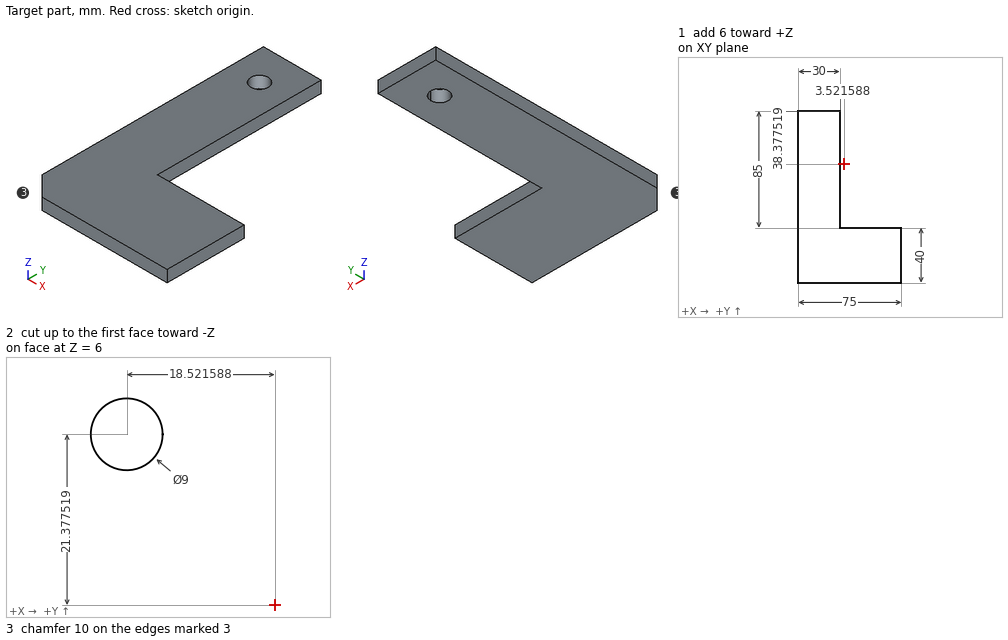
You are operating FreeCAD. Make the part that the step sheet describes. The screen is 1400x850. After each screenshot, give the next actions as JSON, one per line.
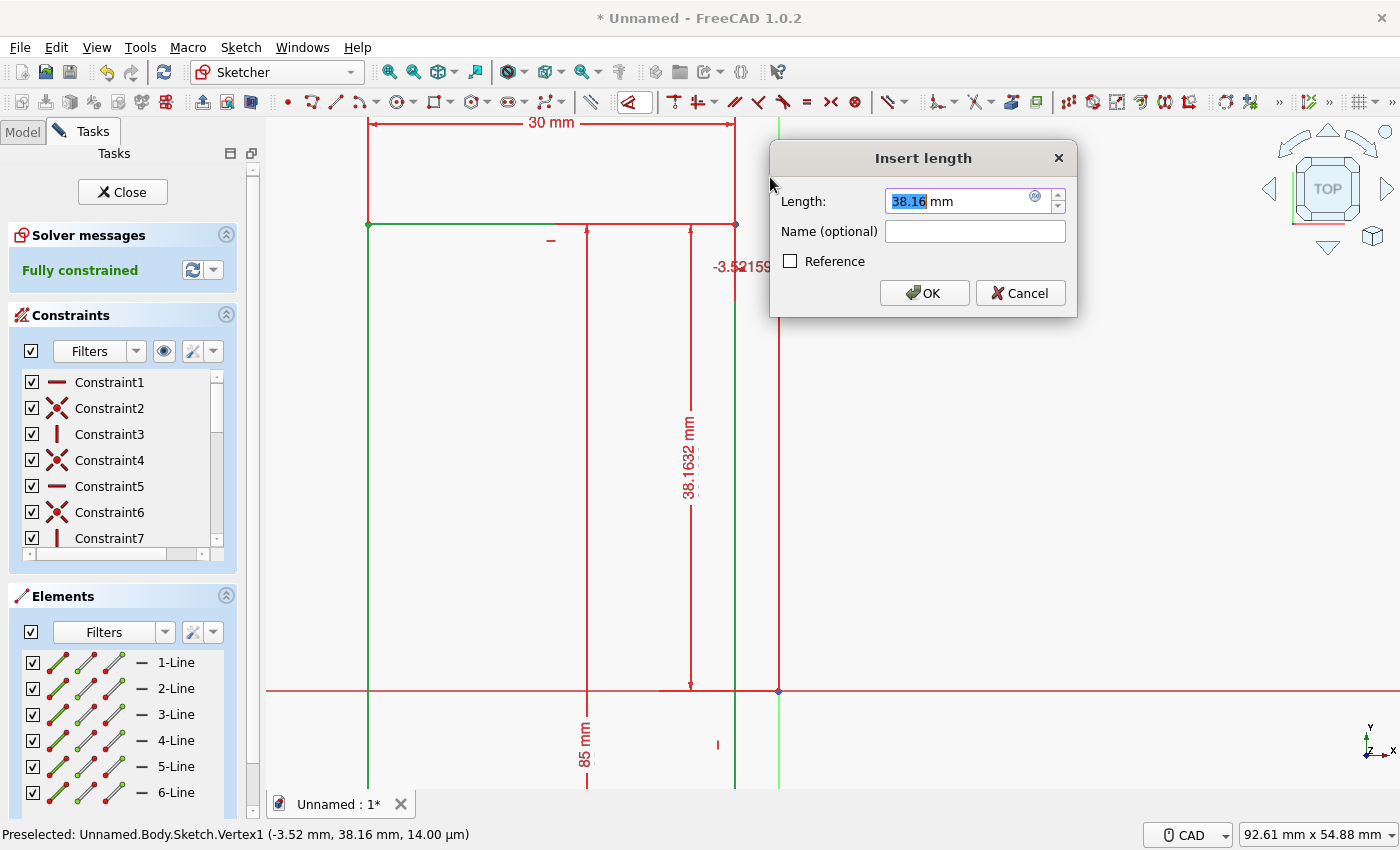
{"action": "type", "text": "38.377519"}
{"action": "key", "text": "Return"}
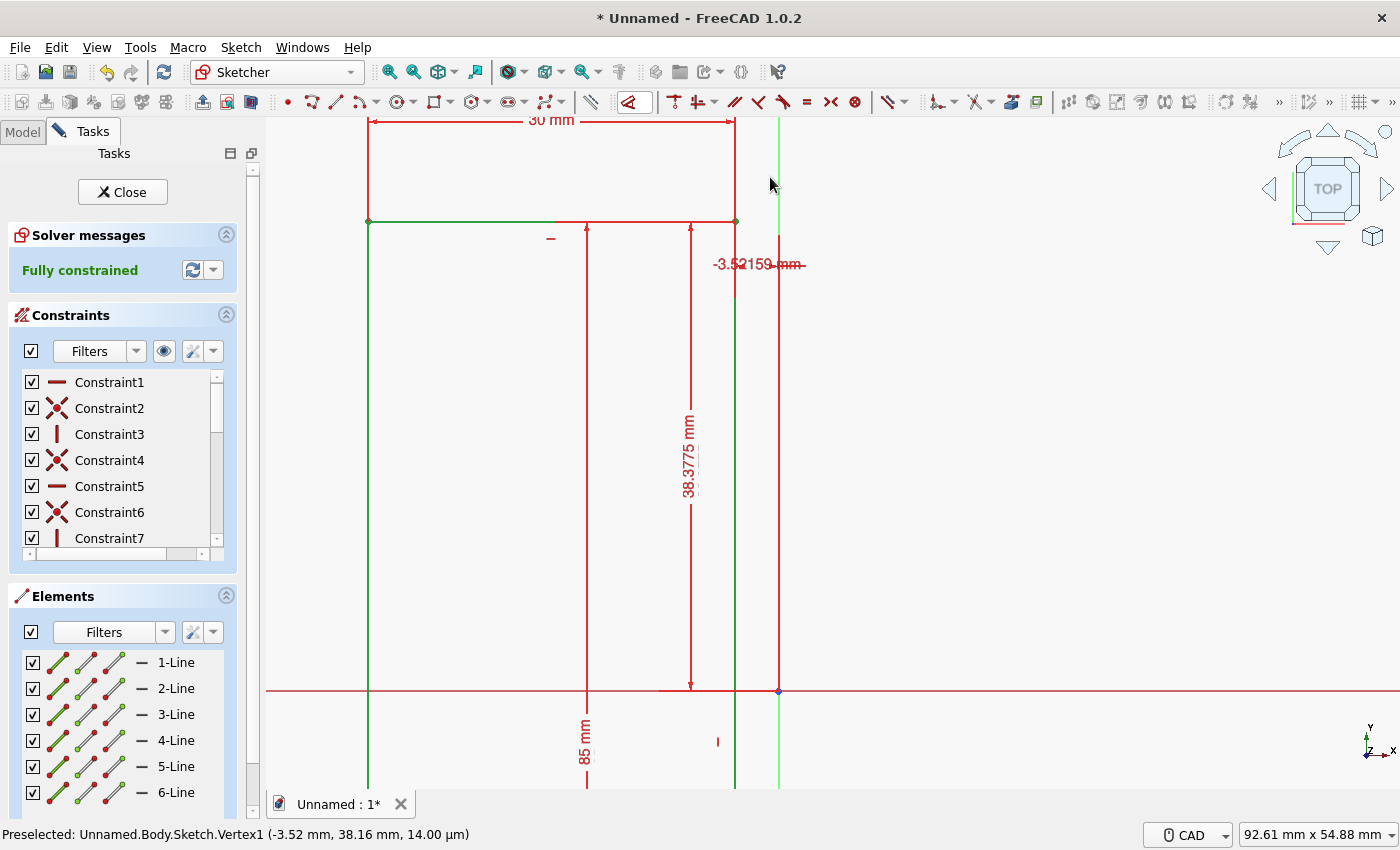
{"action": "left_click", "coordinate": [123, 192]}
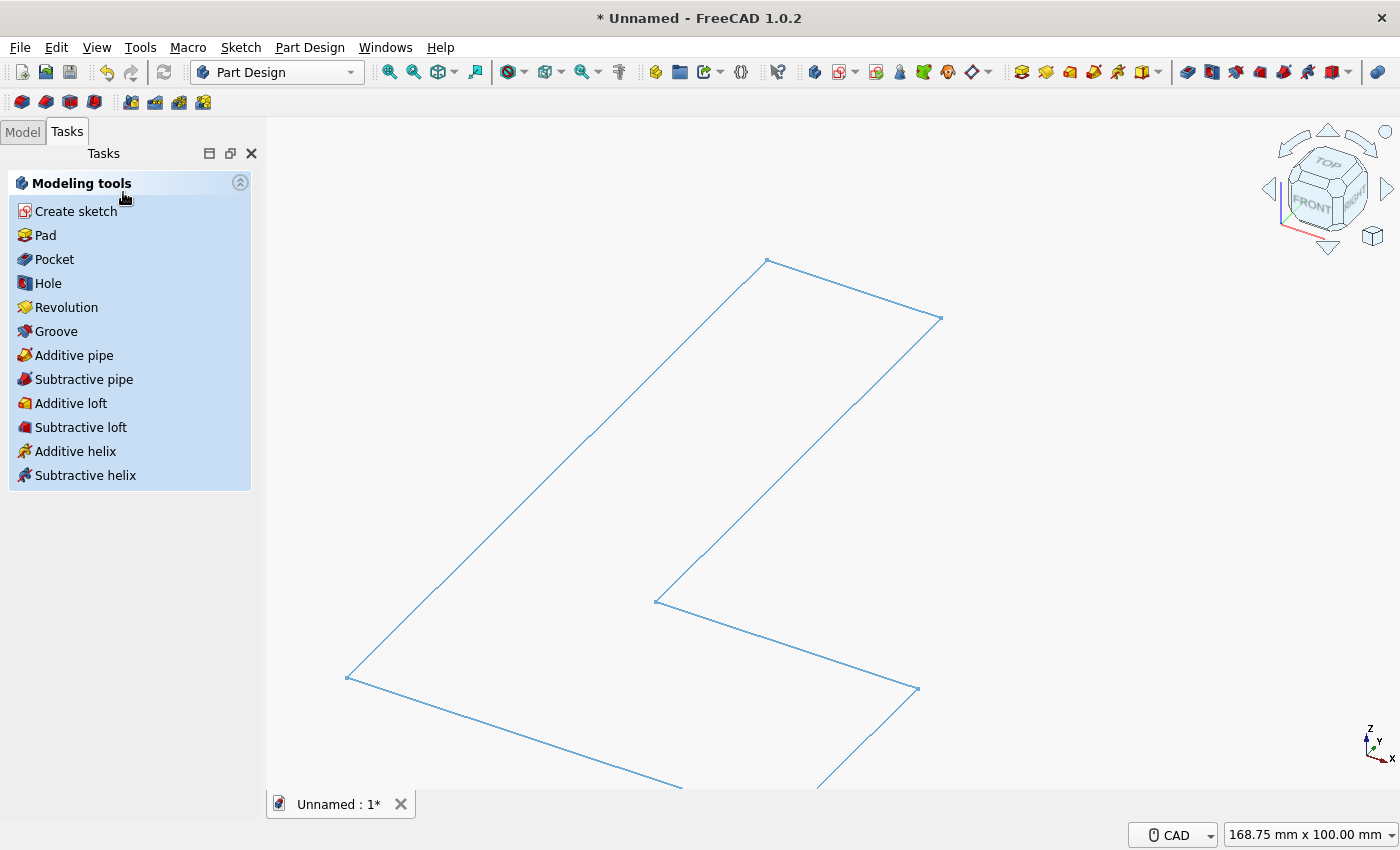
{"action": "left_click", "coordinate": [1022, 72]}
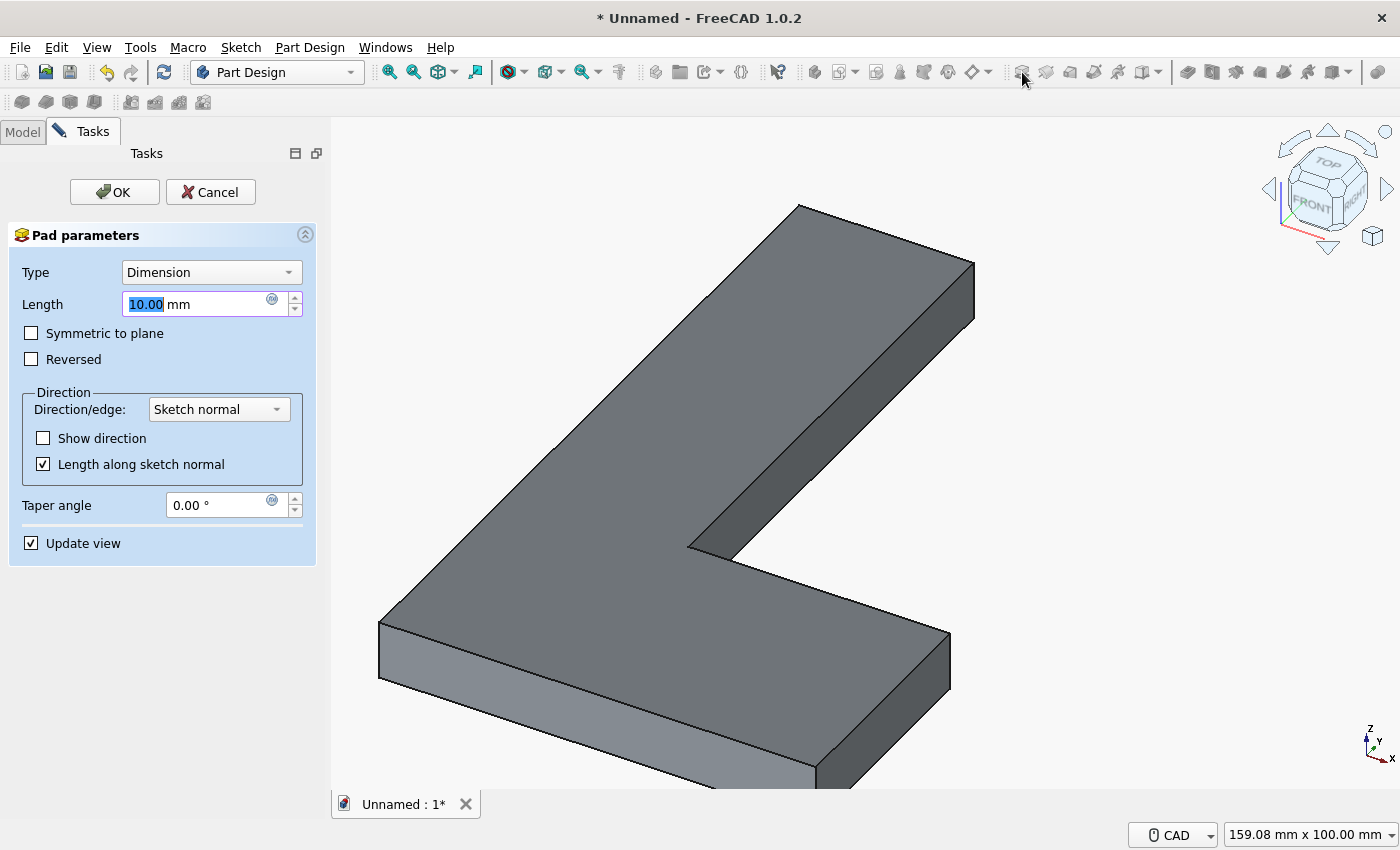
{"action": "type", "text": "6"}
{"action": "key", "text": "Tab"}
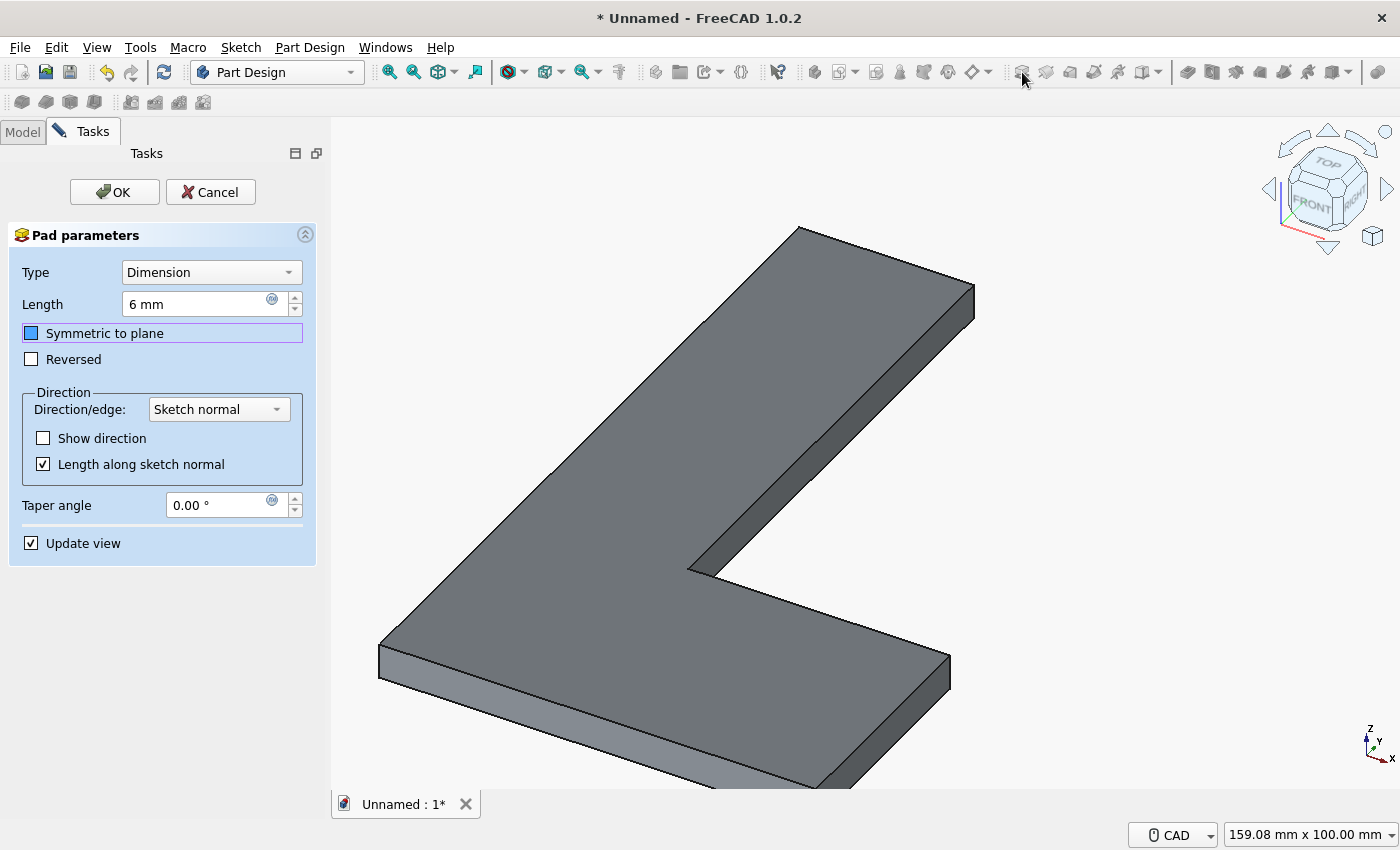
{"action": "left_click", "coordinate": [115, 192]}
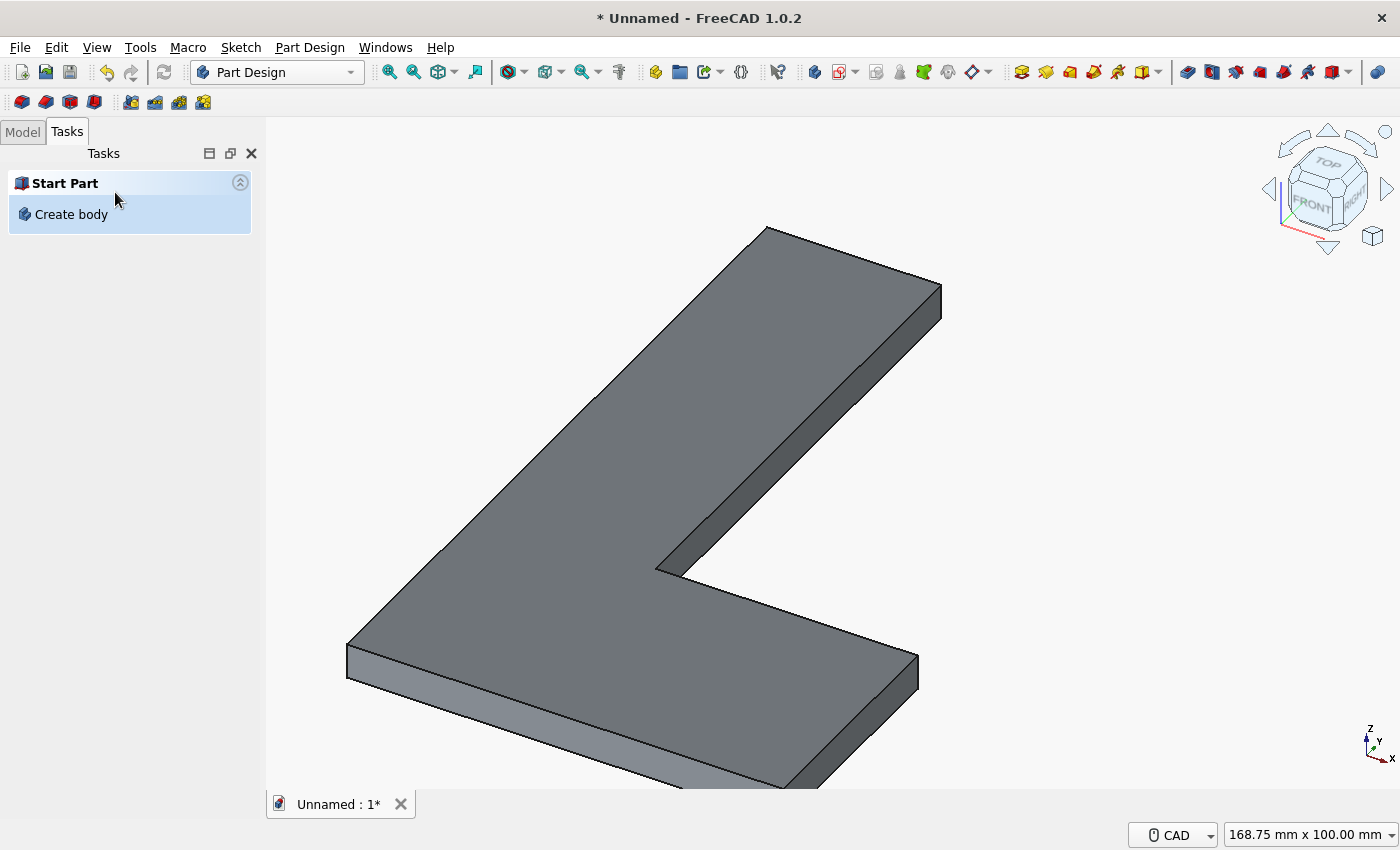
{"action": "left_click", "coordinate": [390, 72]}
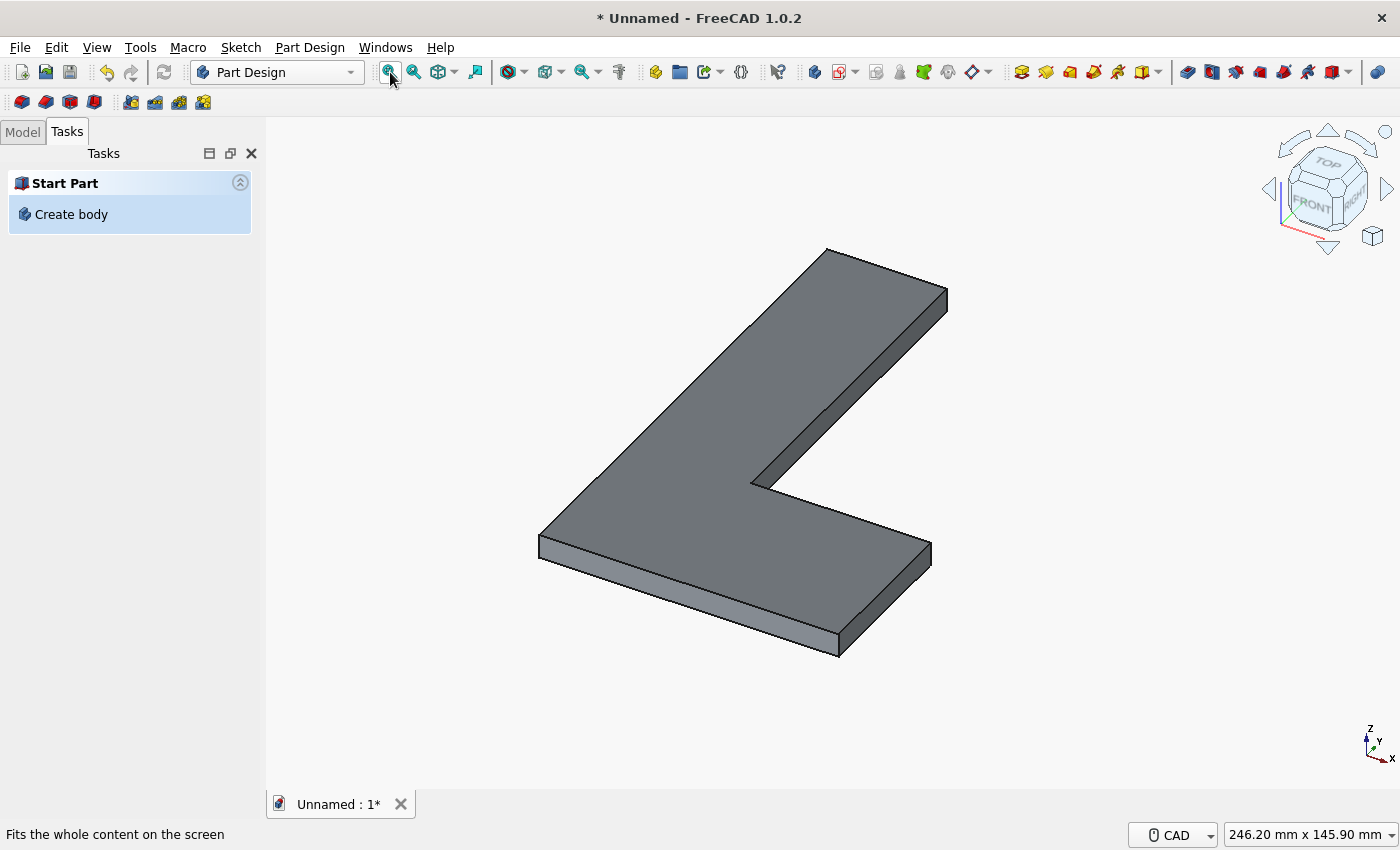
{"action": "left_click", "coordinate": [665, 494]}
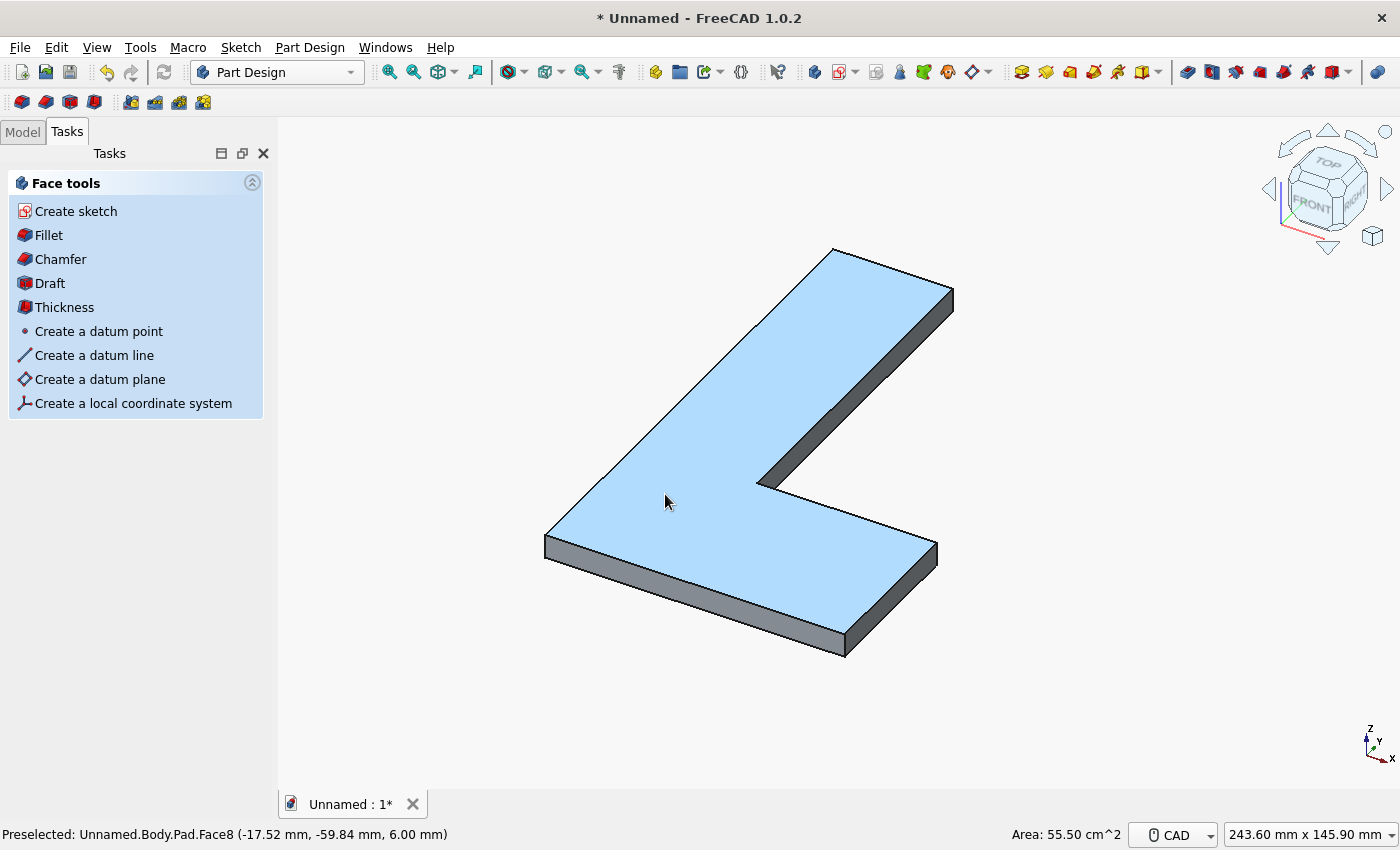
{"action": "left_click", "coordinate": [840, 72]}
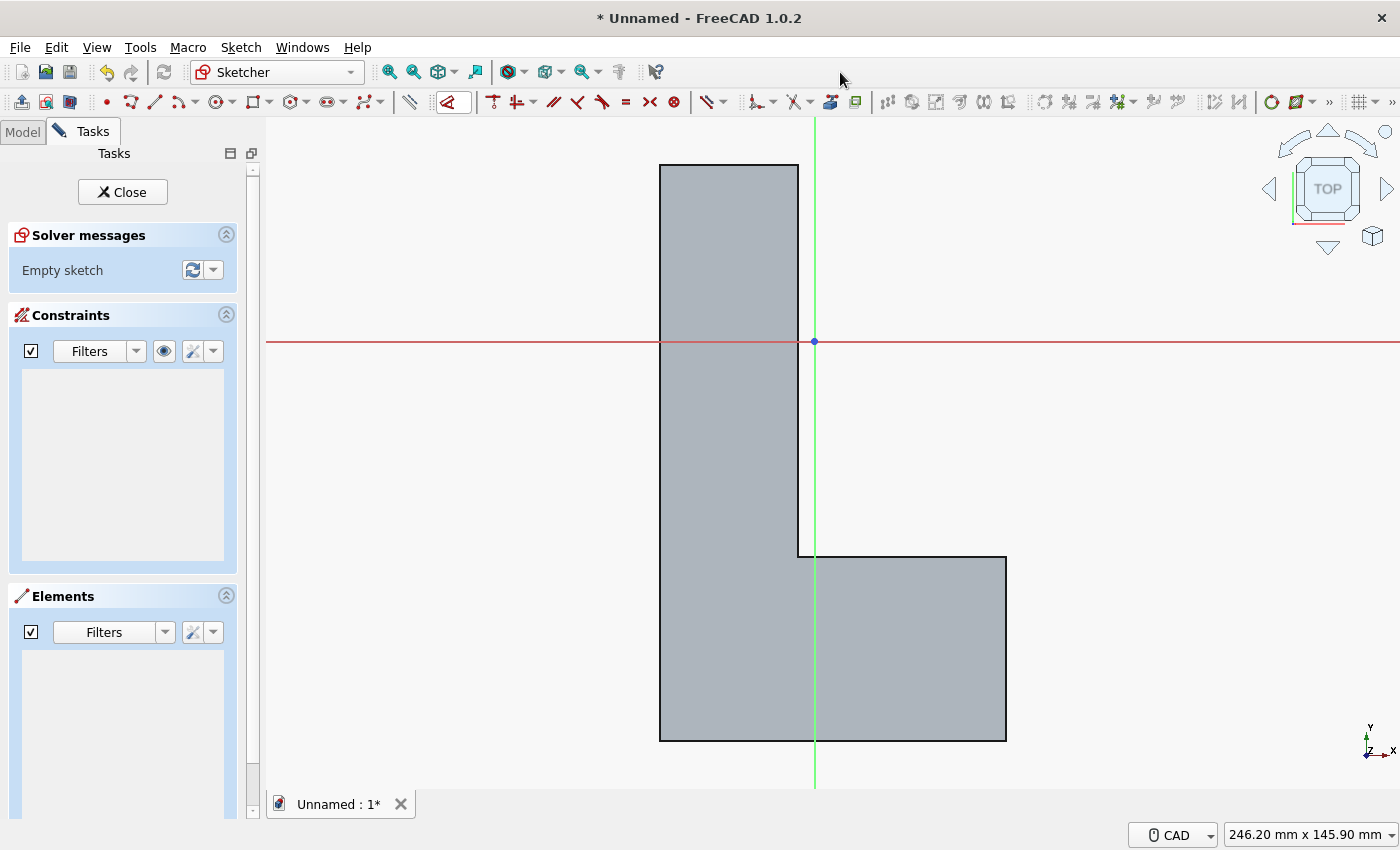
{"action": "scroll", "coordinate": [726, 223], "scroll_direction": "up", "scroll_amount": 12}